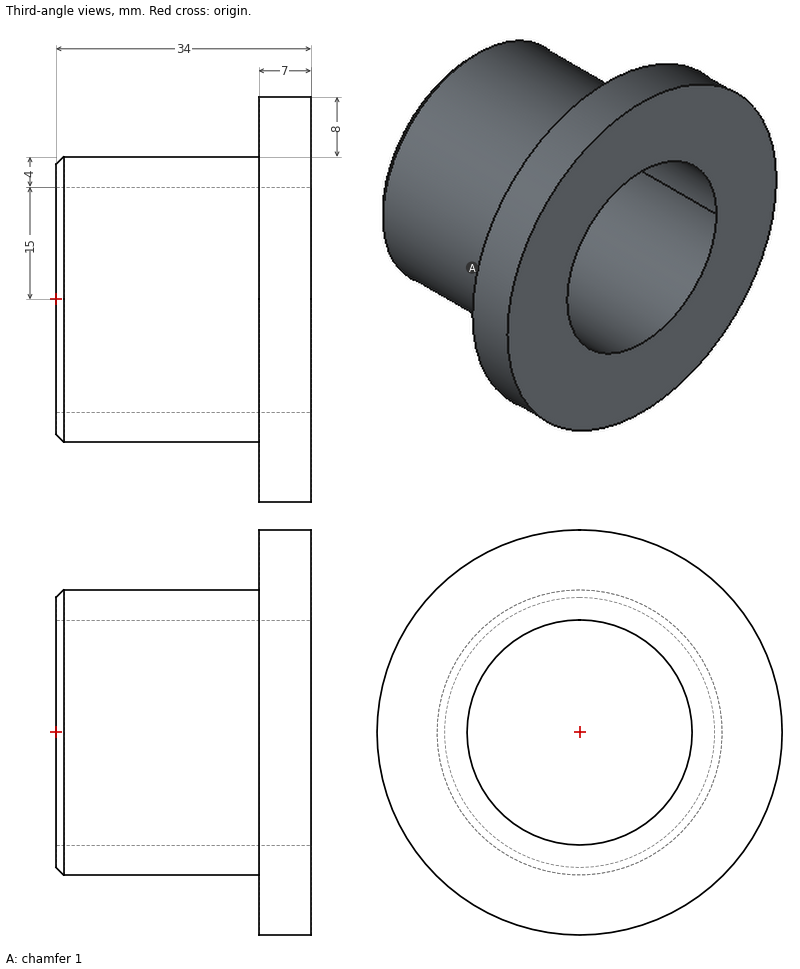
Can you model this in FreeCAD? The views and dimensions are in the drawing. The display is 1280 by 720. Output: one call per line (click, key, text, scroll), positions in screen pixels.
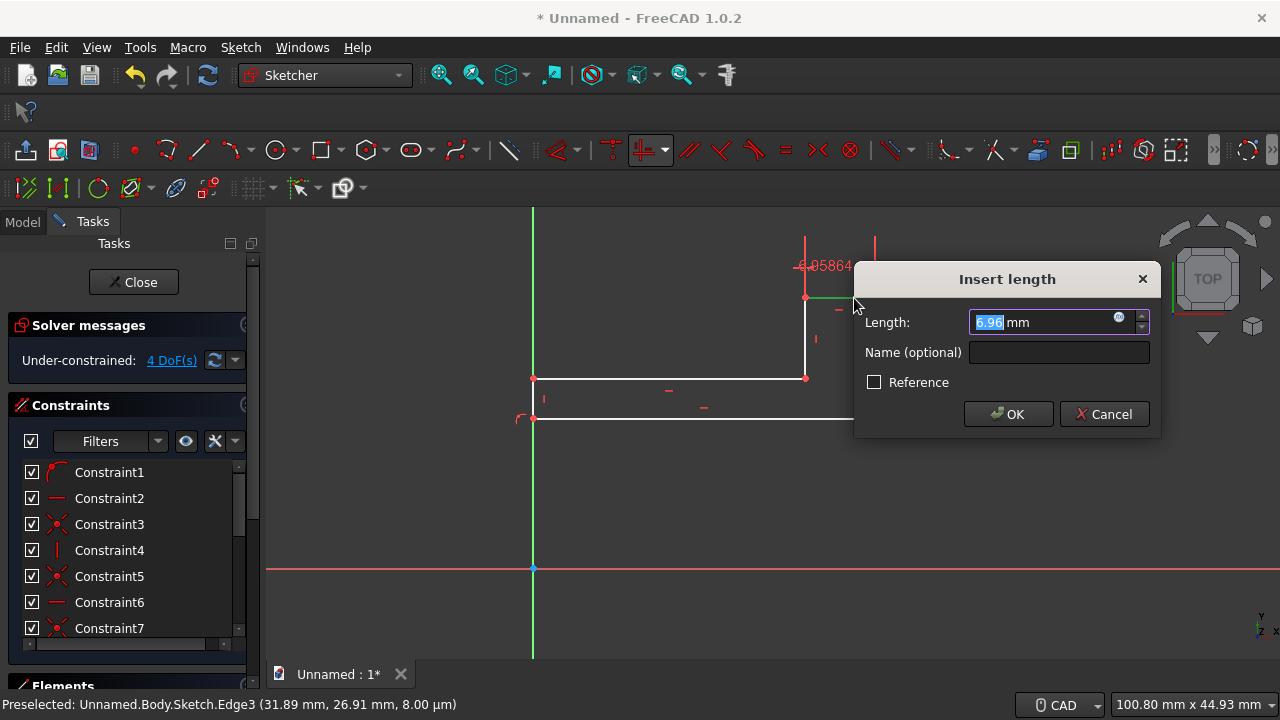
text(7)
key(Return)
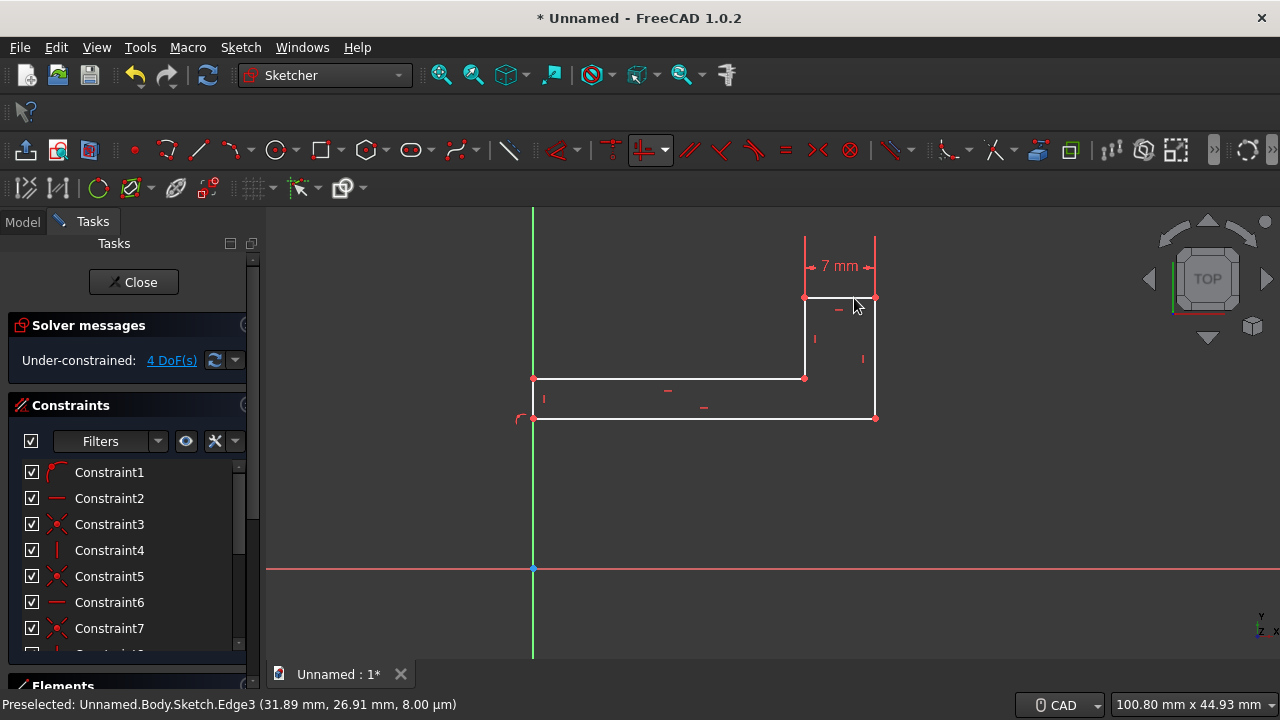
click(805, 322)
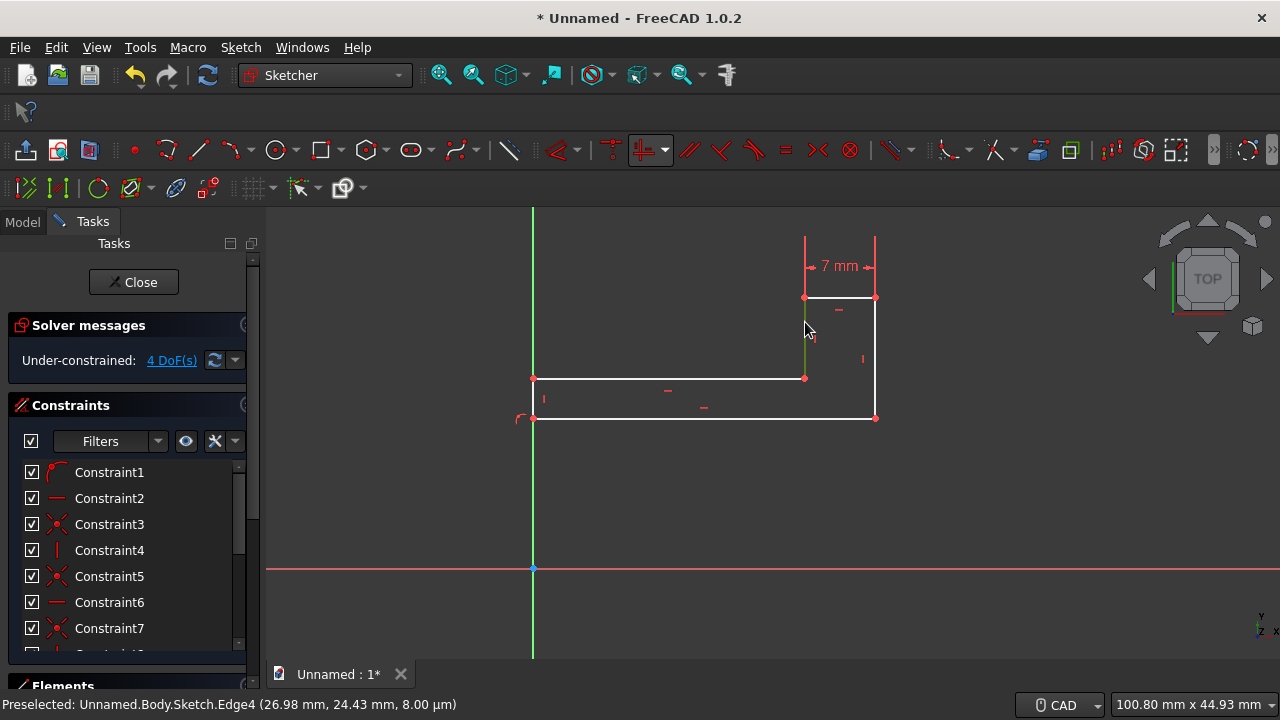
key(i)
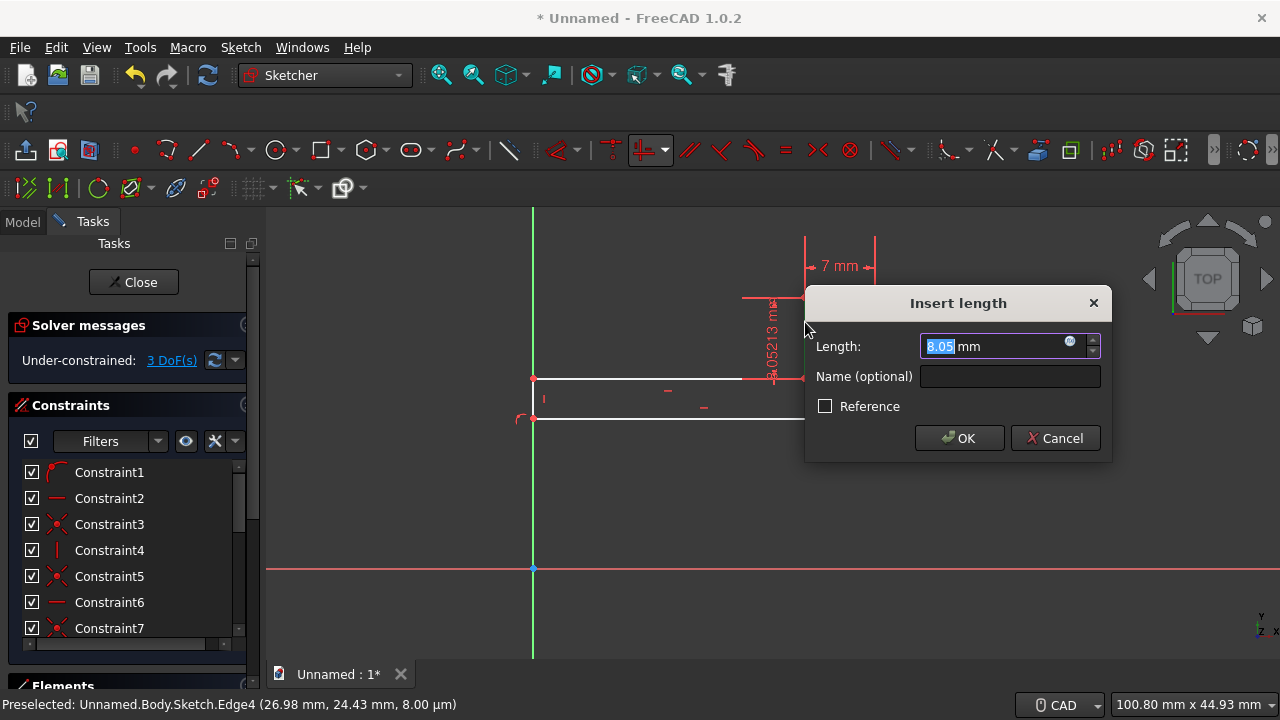
text(8)
key(Return)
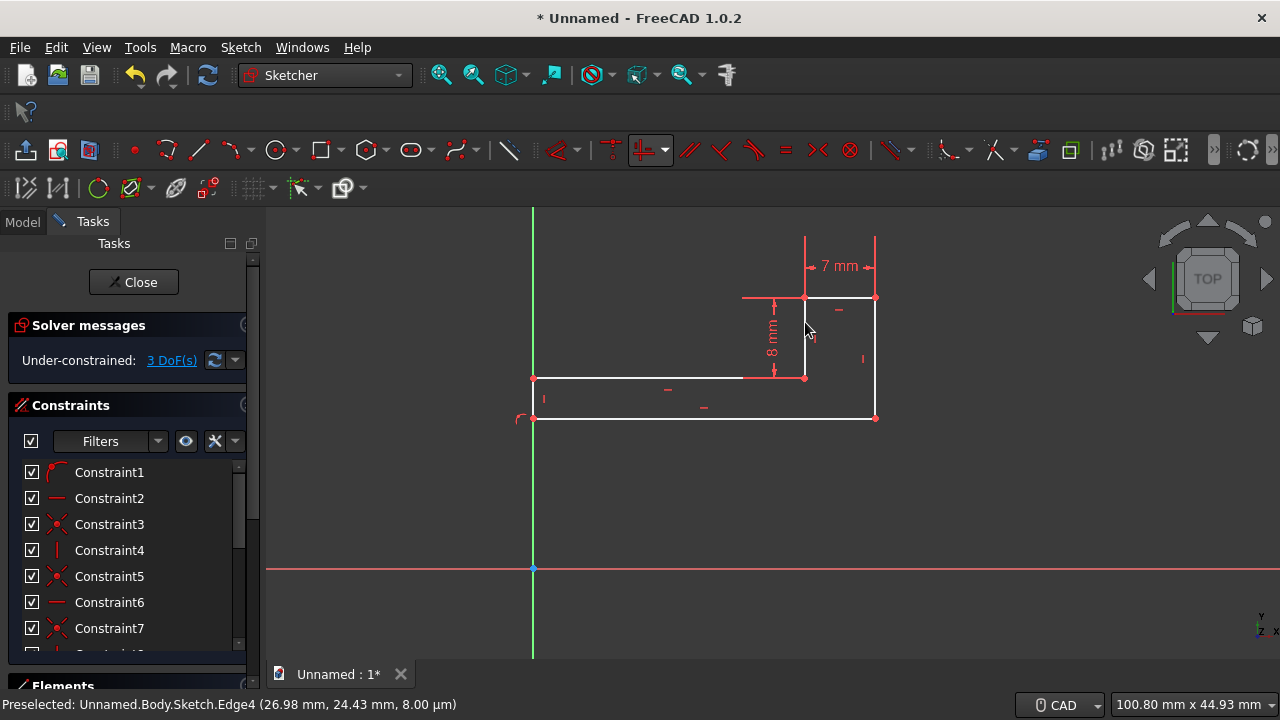
click(533, 391)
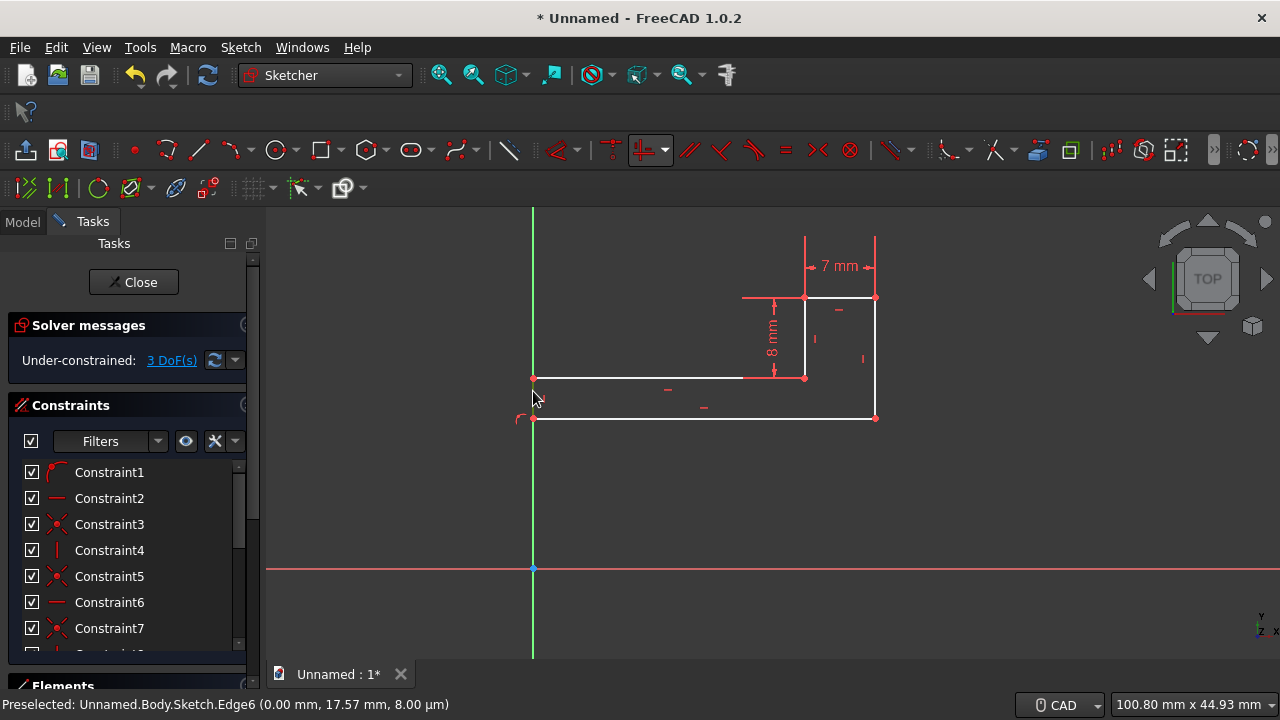
click(580, 150)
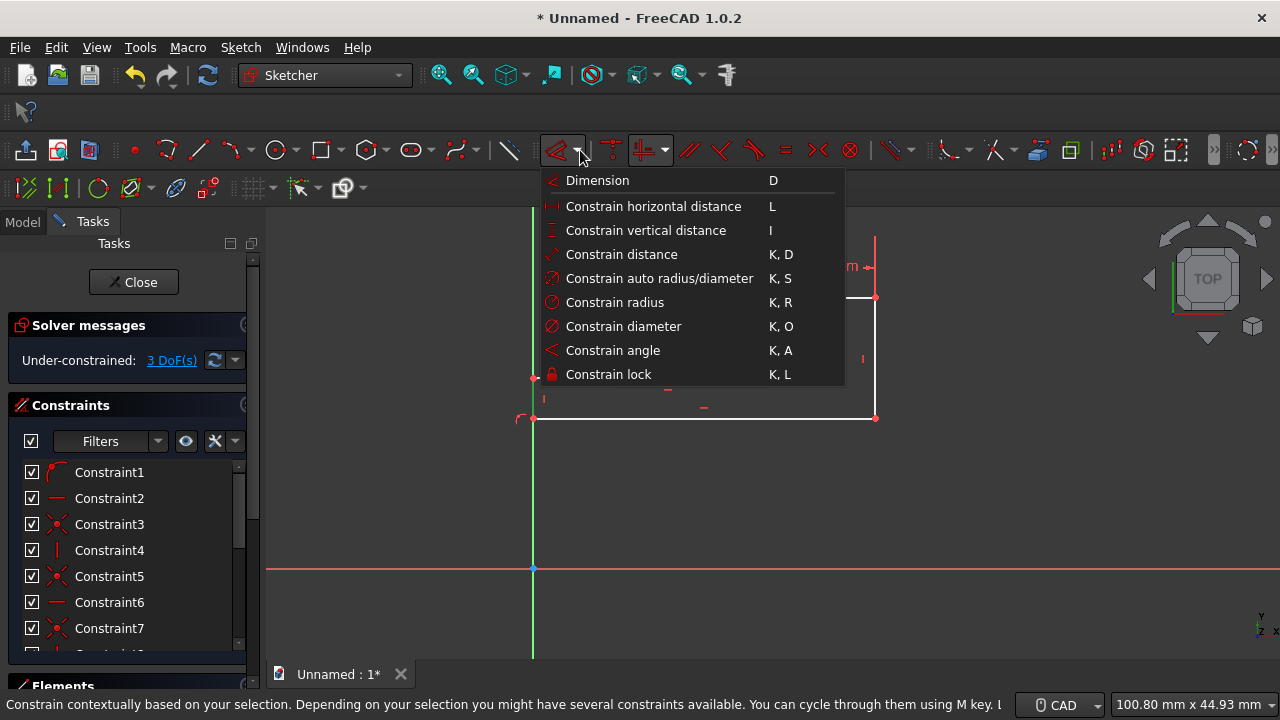
click(693, 230)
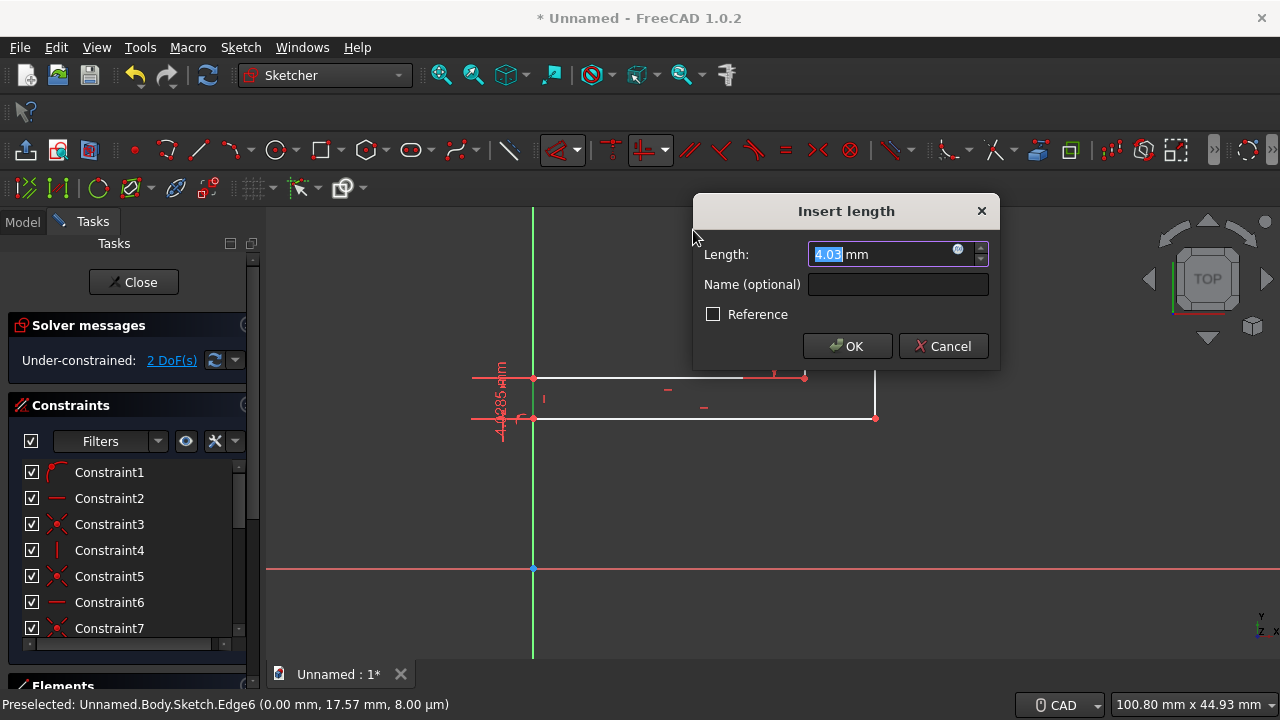
text(4)
key(Return)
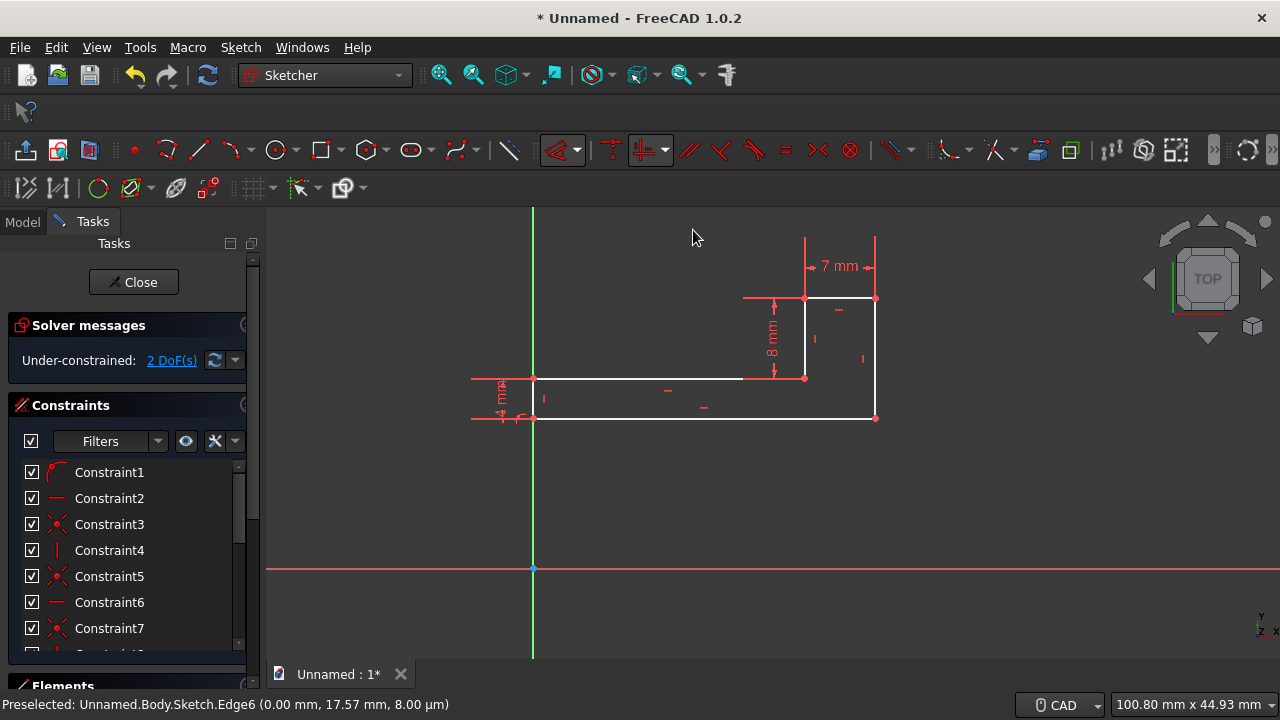
click(636, 419)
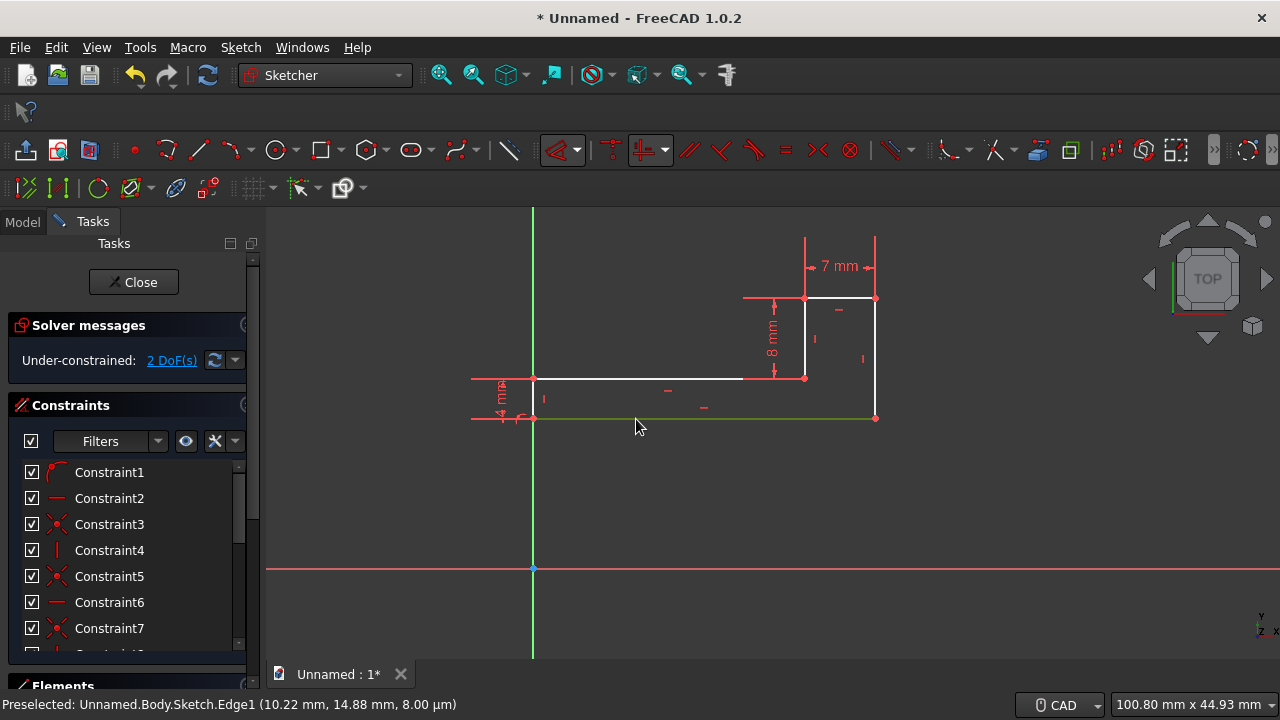
key(l)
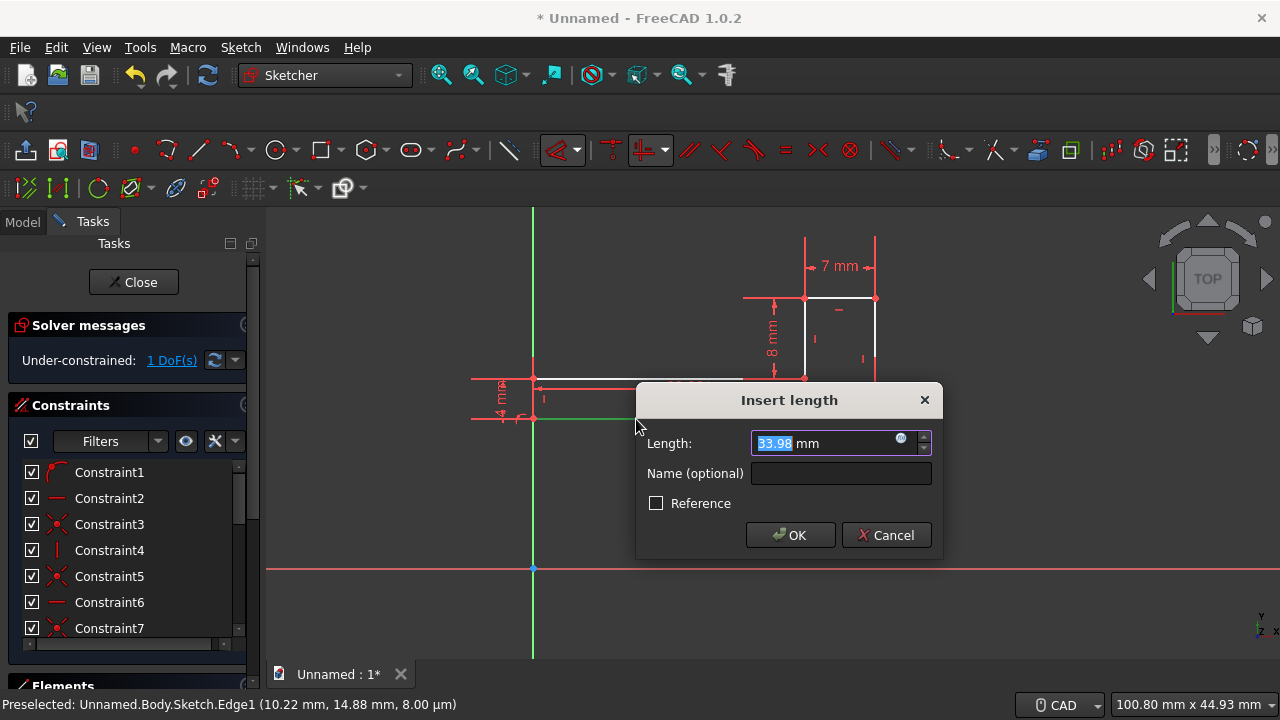
text(34)
key(Return)